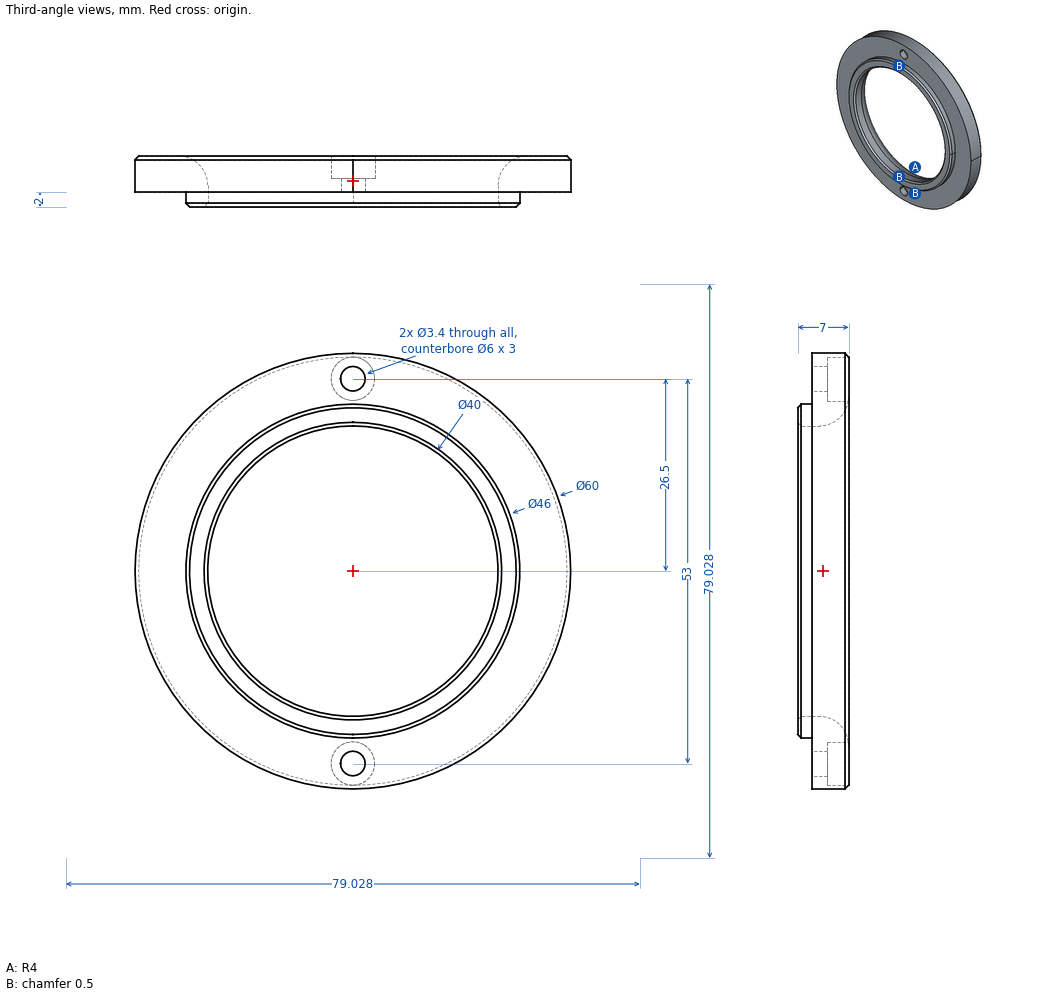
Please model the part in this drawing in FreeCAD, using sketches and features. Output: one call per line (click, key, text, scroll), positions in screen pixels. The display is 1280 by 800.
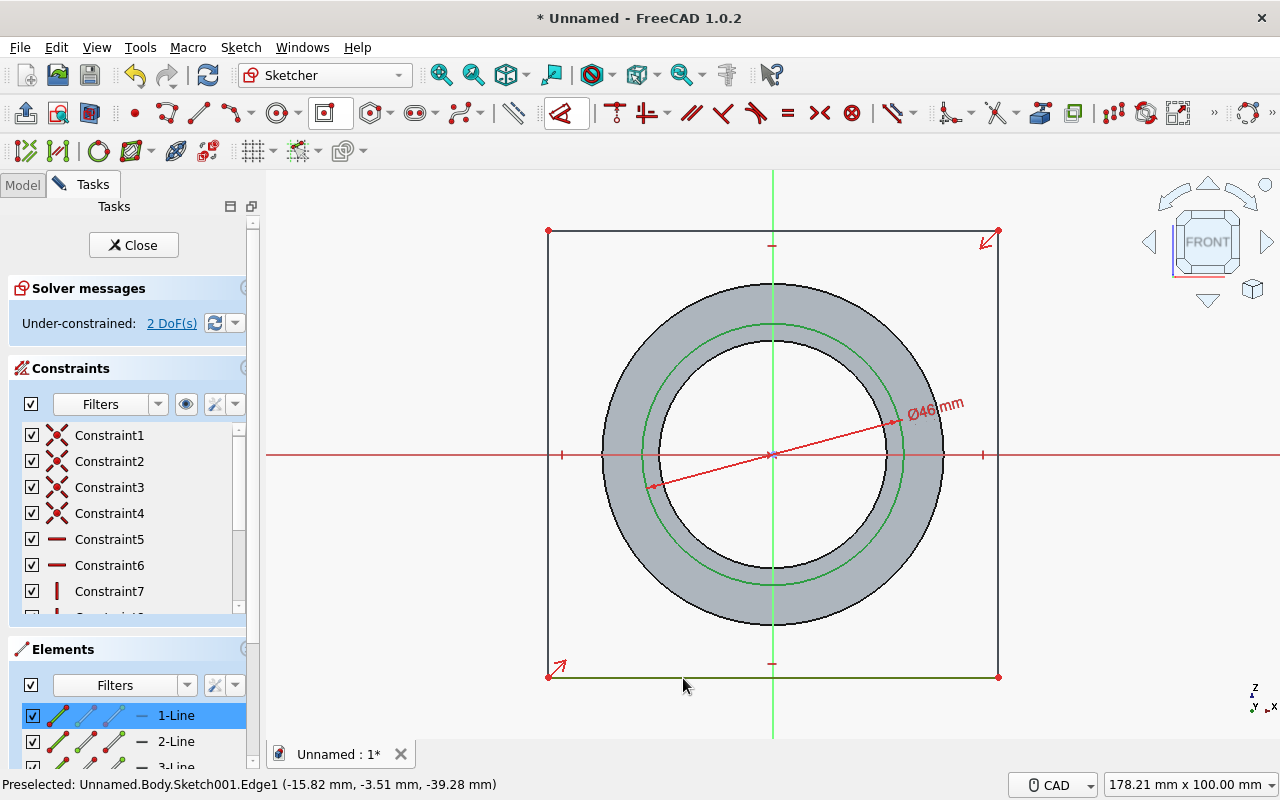
click(584, 114)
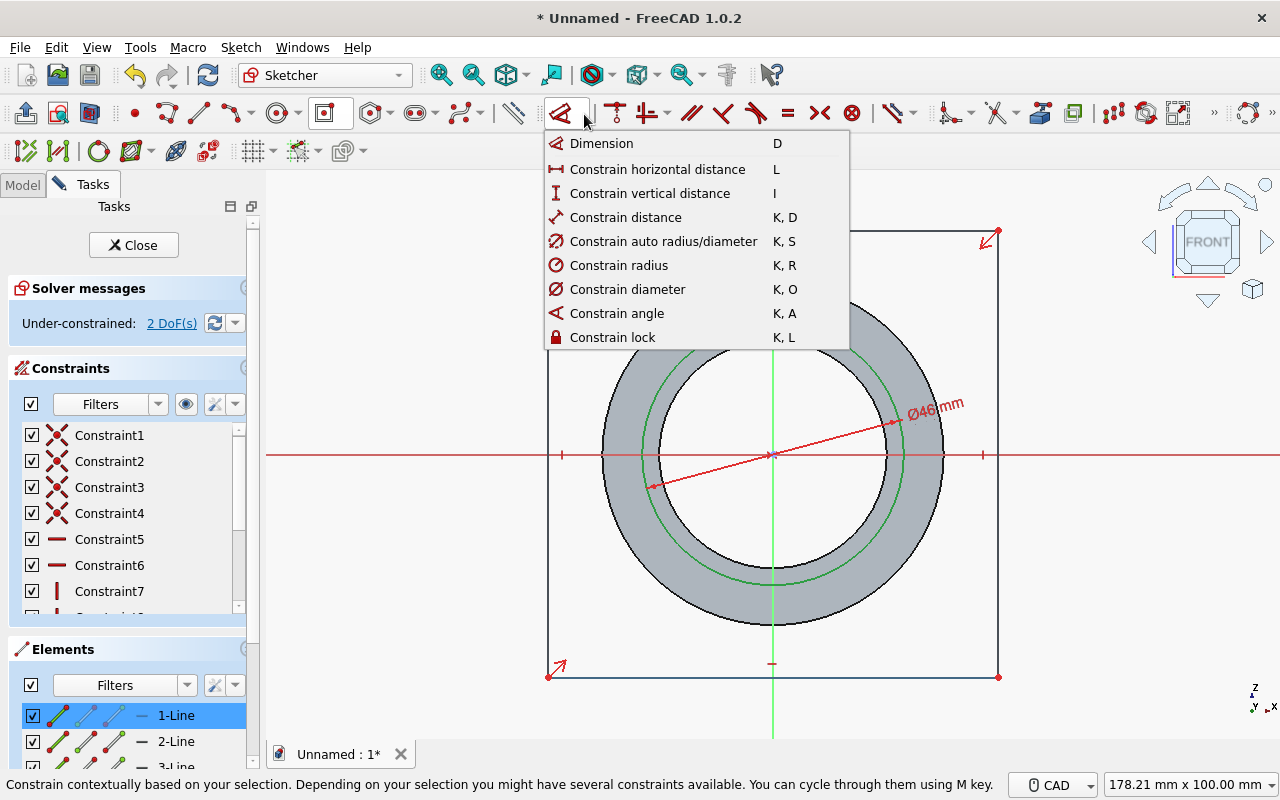
click(697, 169)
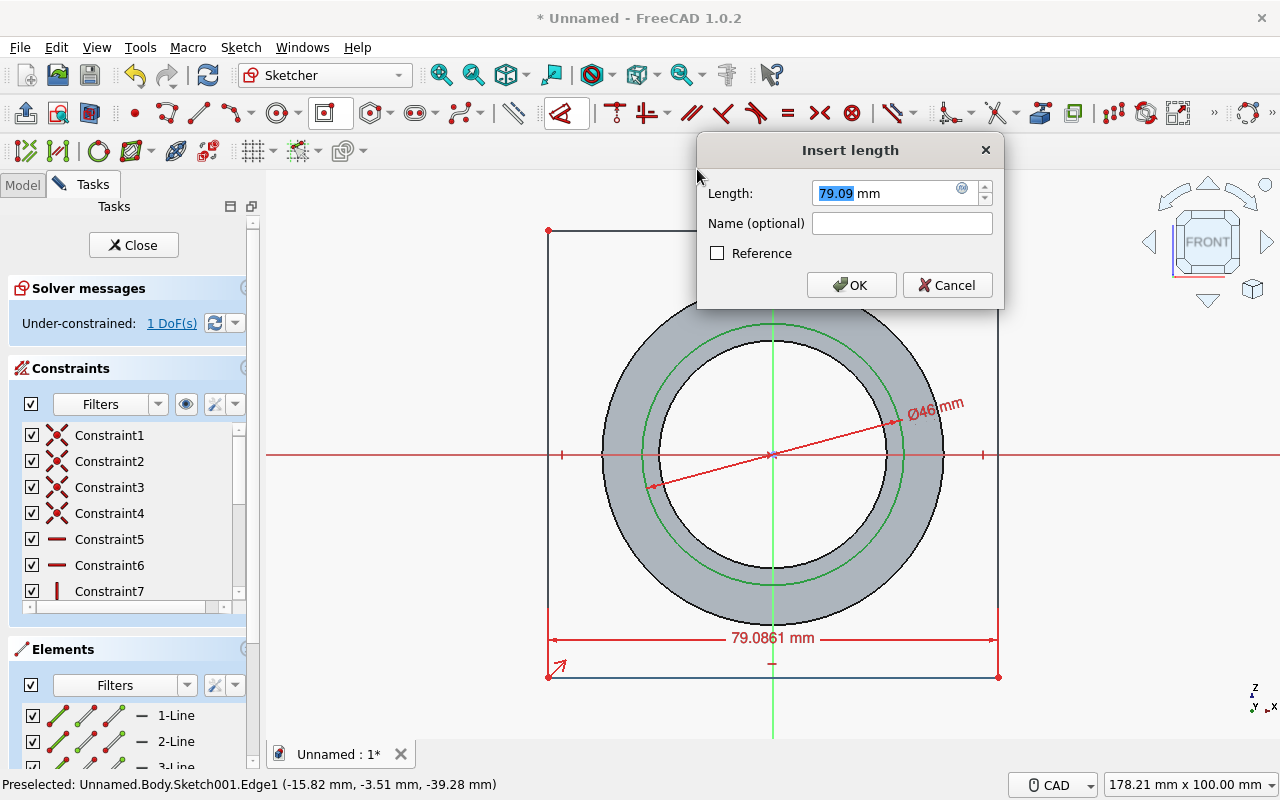
text(79.028)
key(Return)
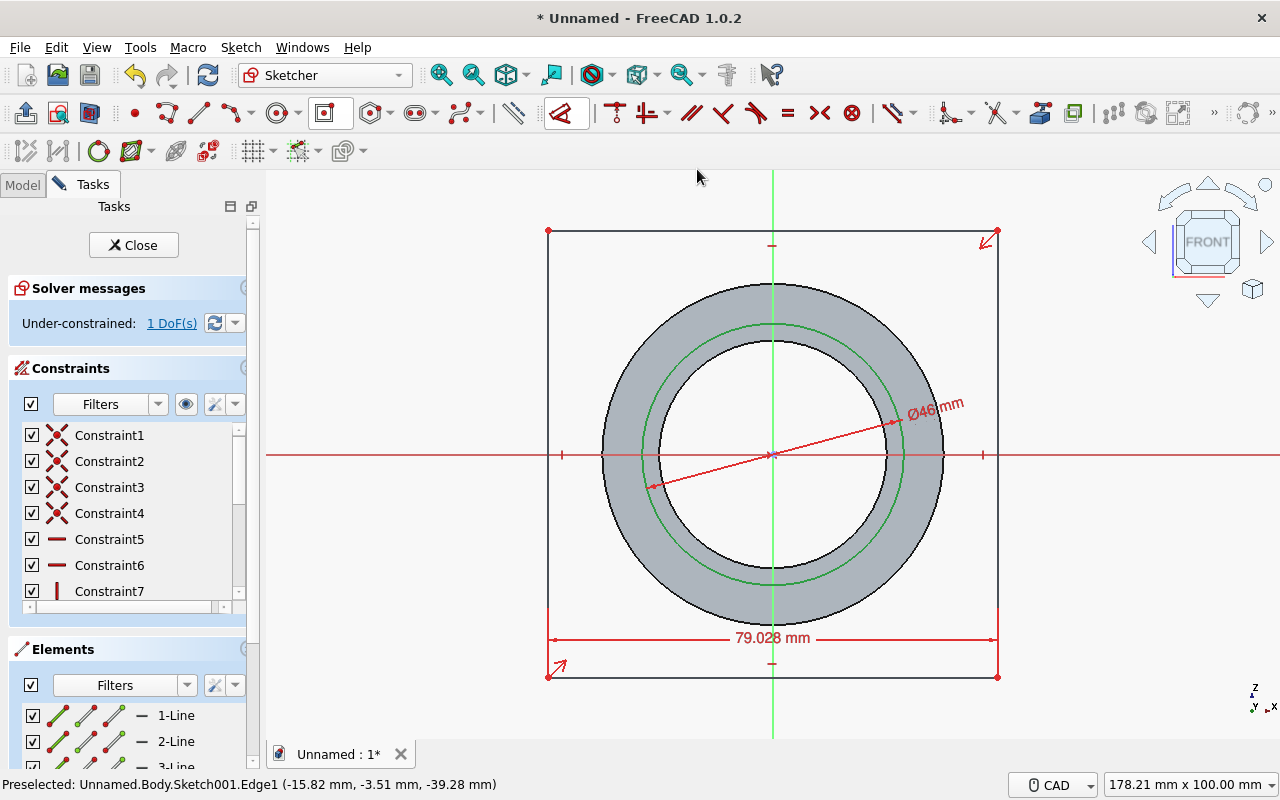
click(998, 544)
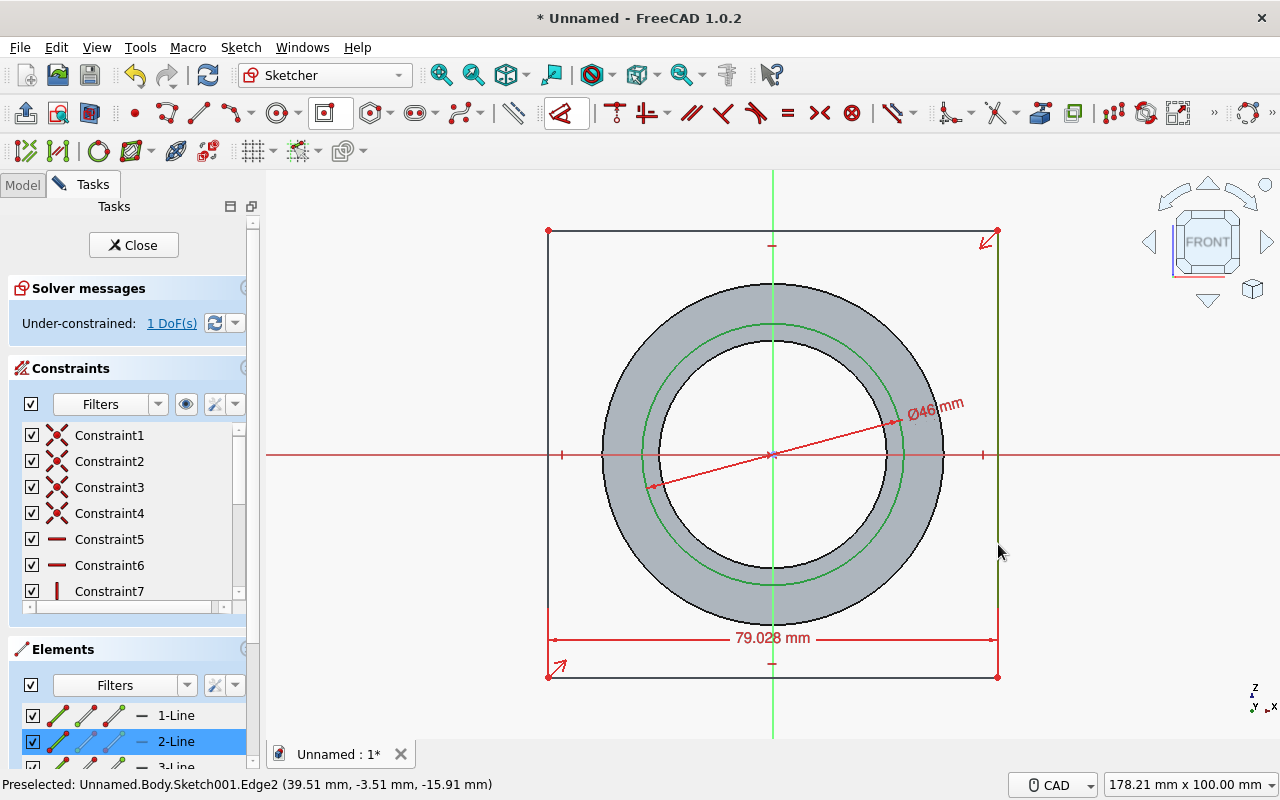
key(i)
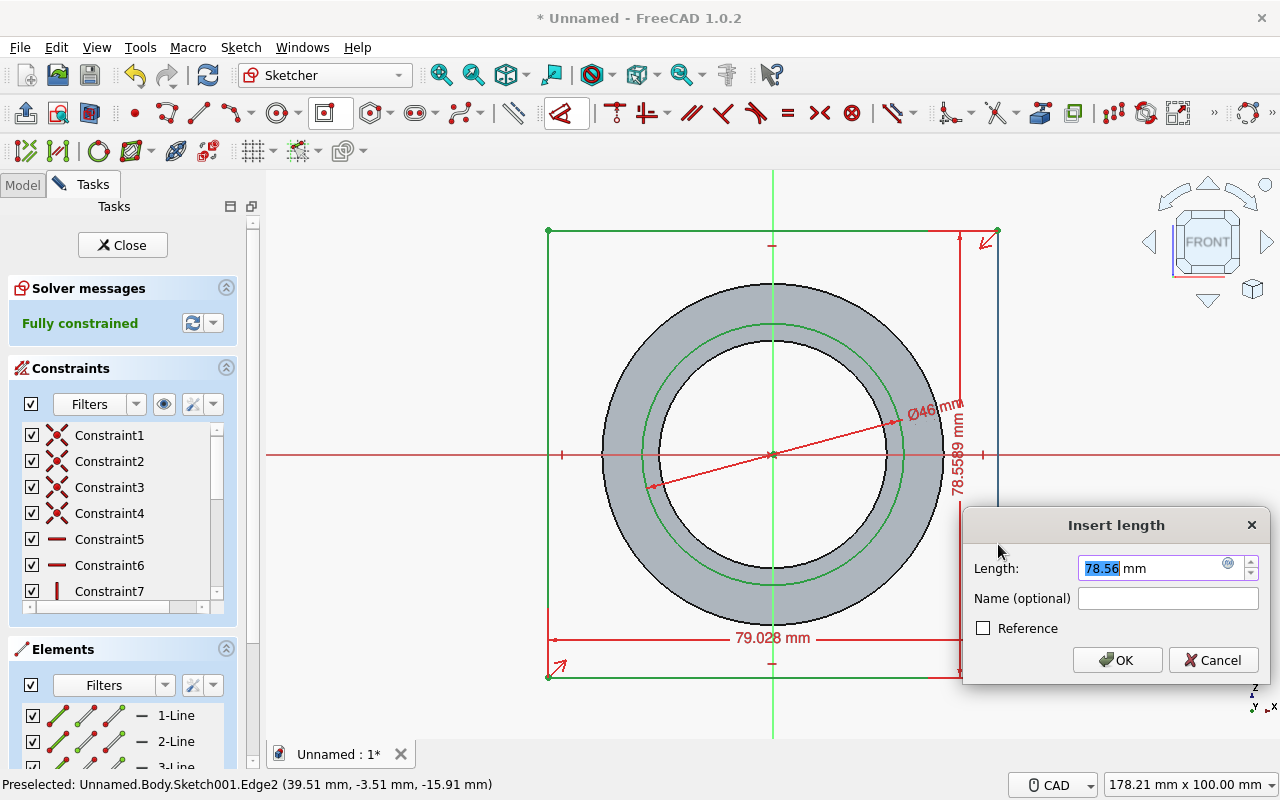
text(79.028)
key(Return)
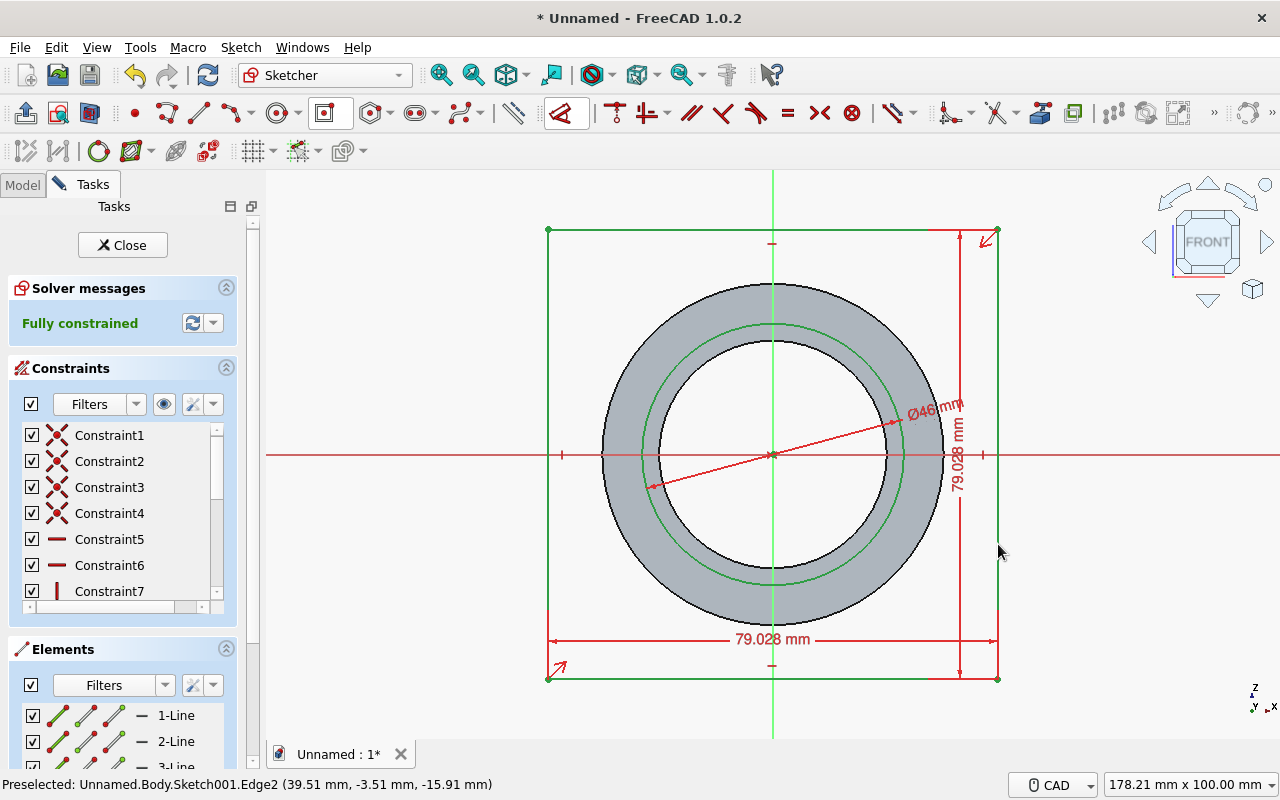
click(123, 245)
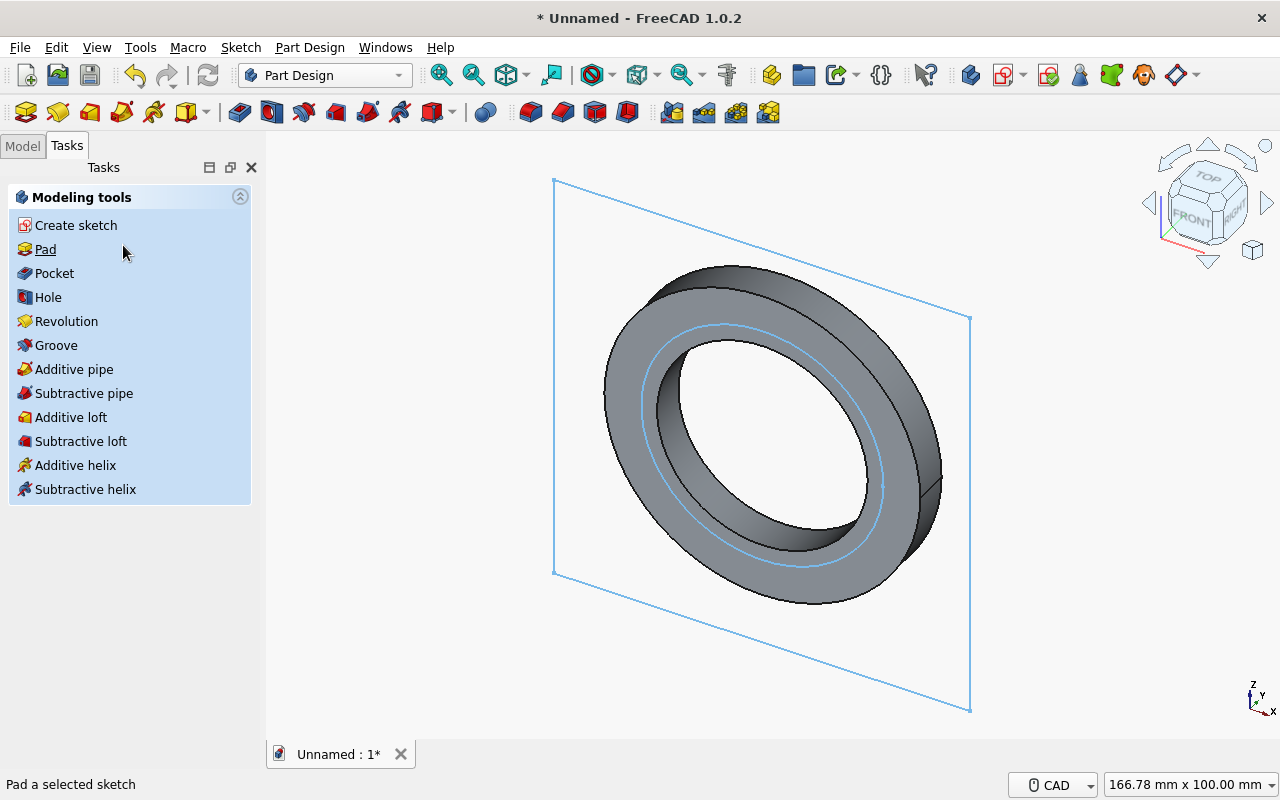
click(240, 112)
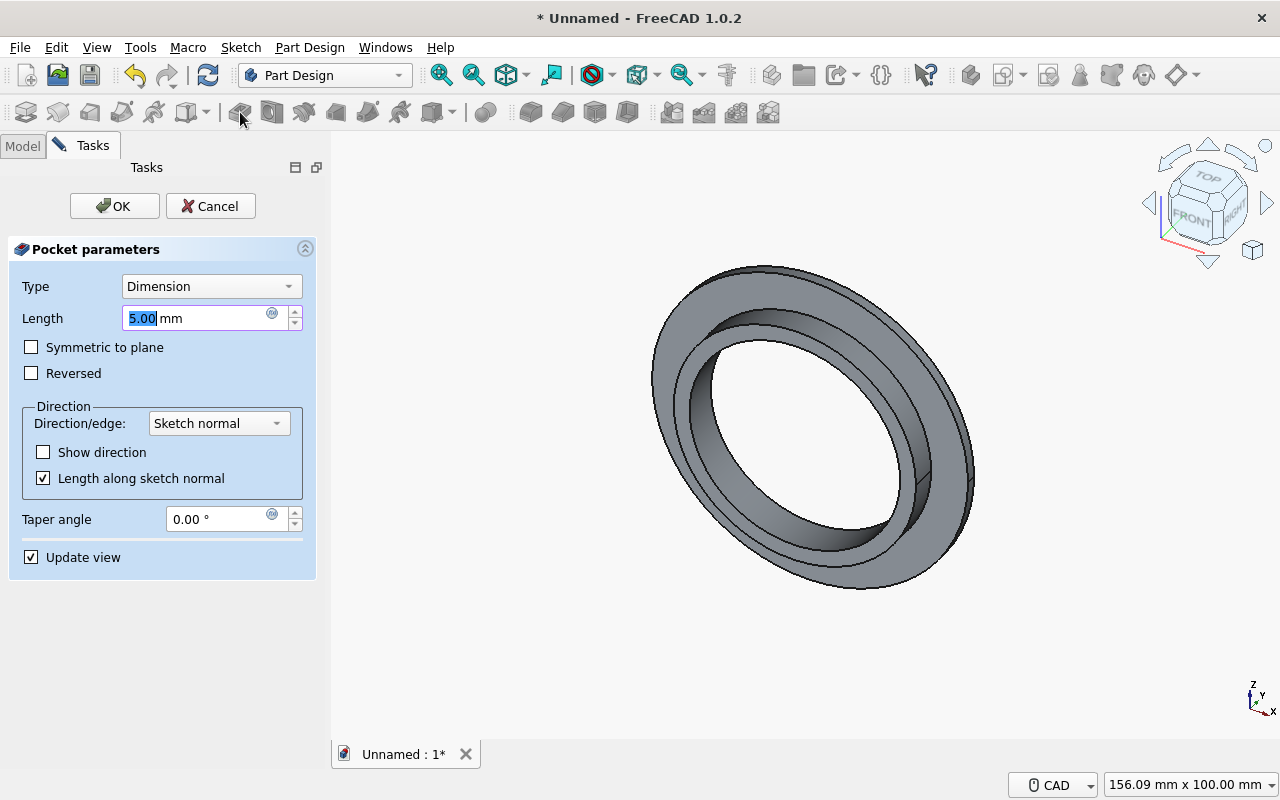
text(2)
key(Tab)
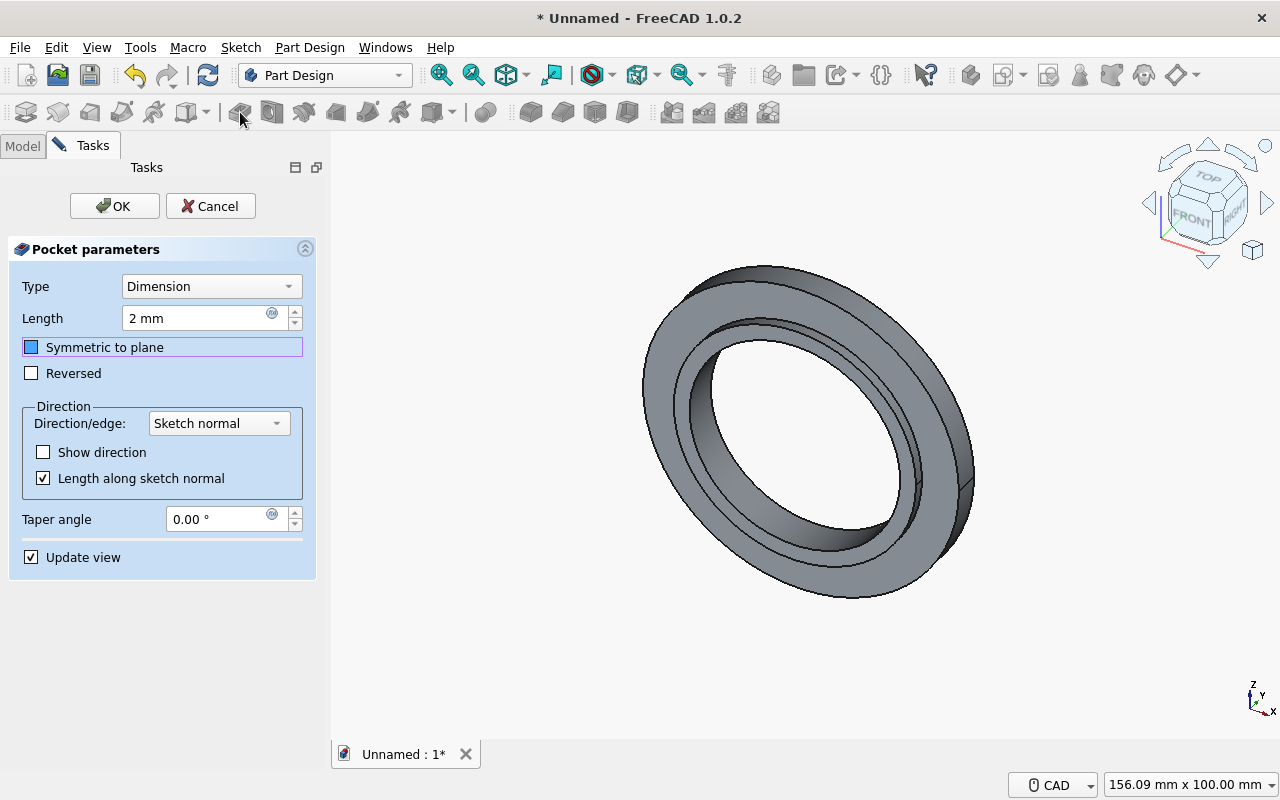
click(115, 206)